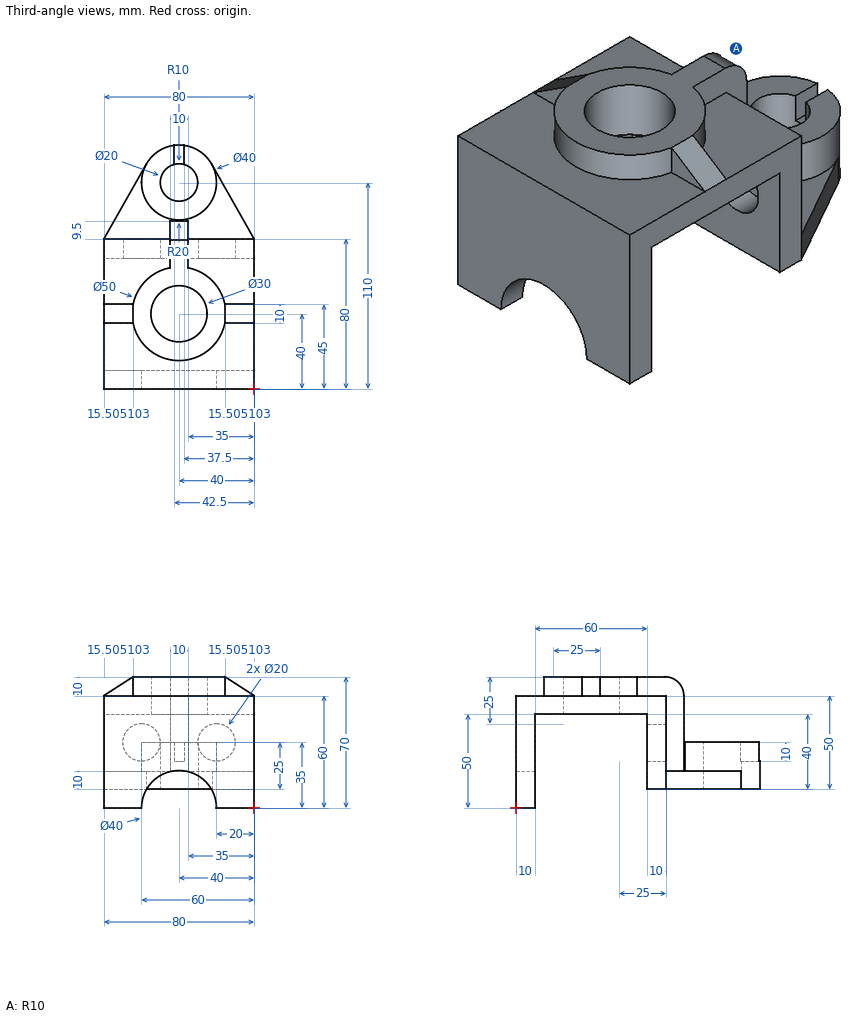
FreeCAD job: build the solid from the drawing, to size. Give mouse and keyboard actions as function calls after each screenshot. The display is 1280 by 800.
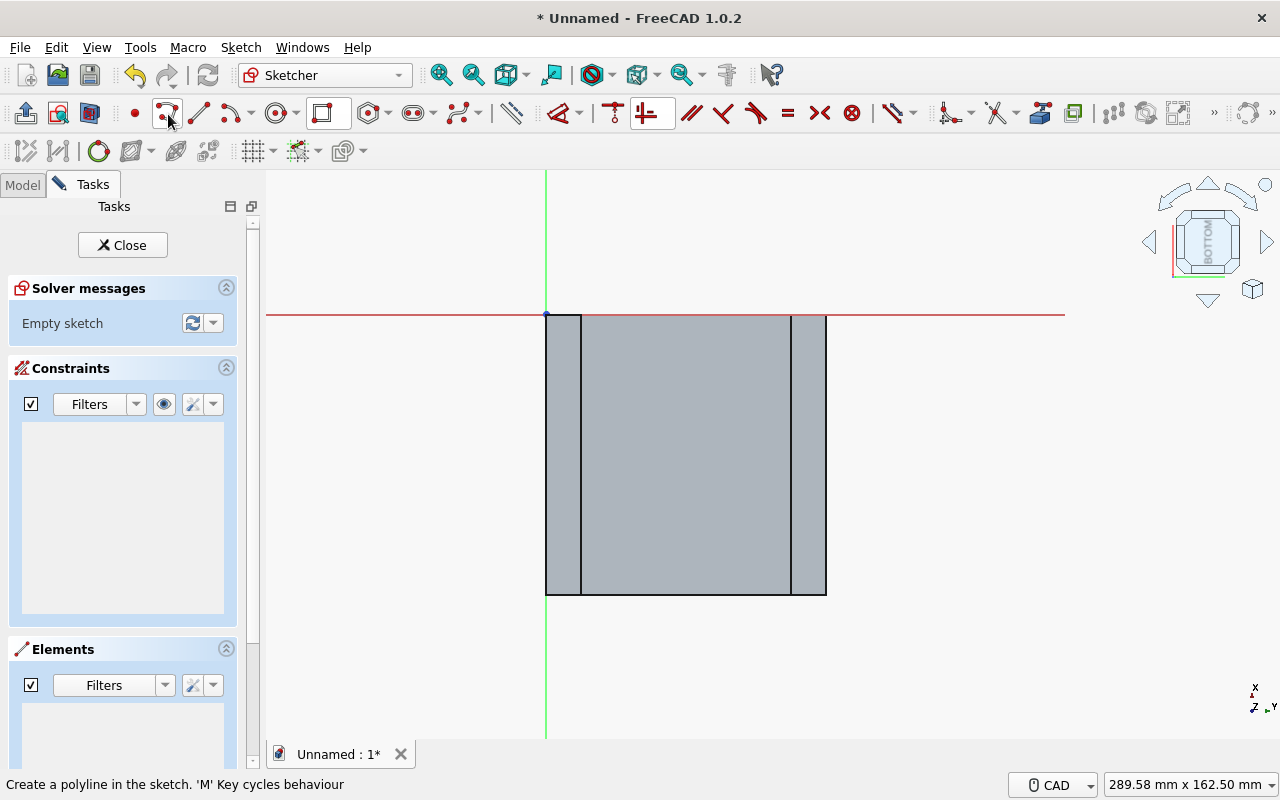
click(966, 394)
click(826, 315)
click(826, 595)
click(966, 516)
right_click(966, 516)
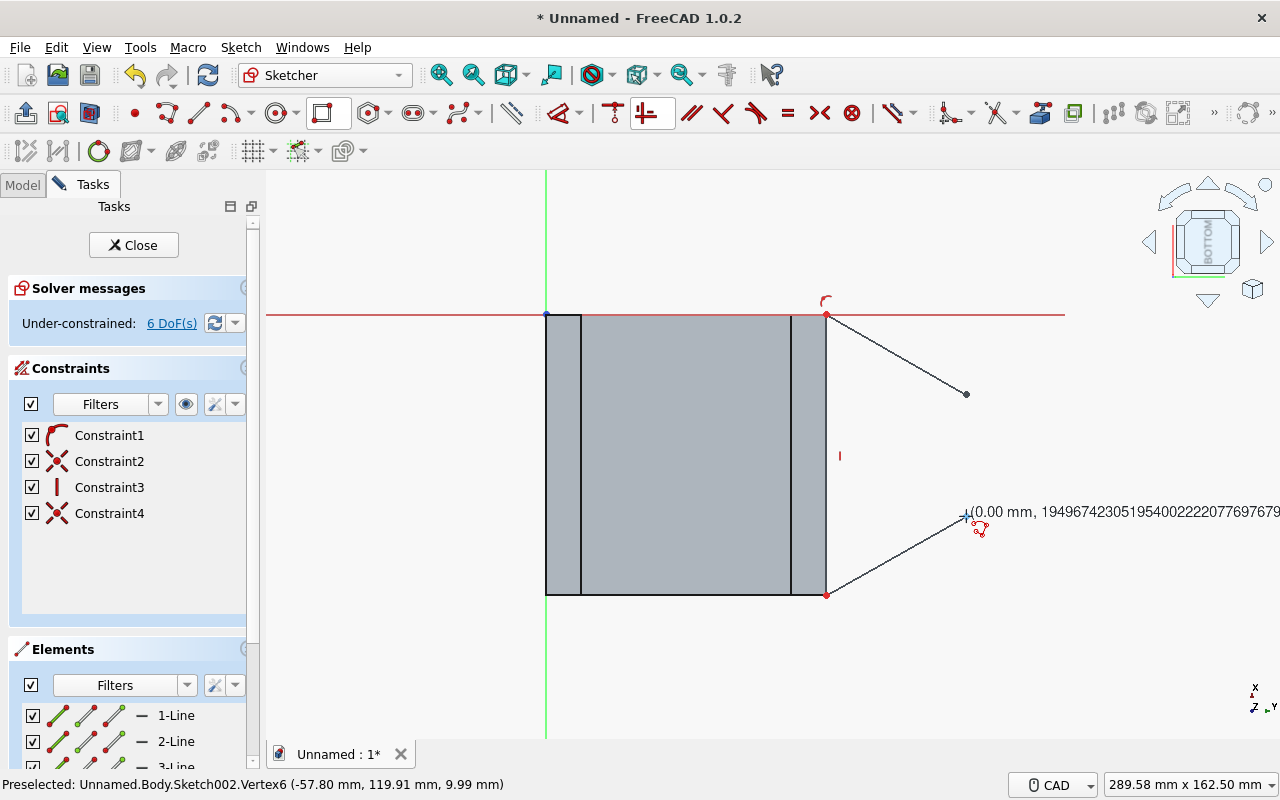
click(254, 114)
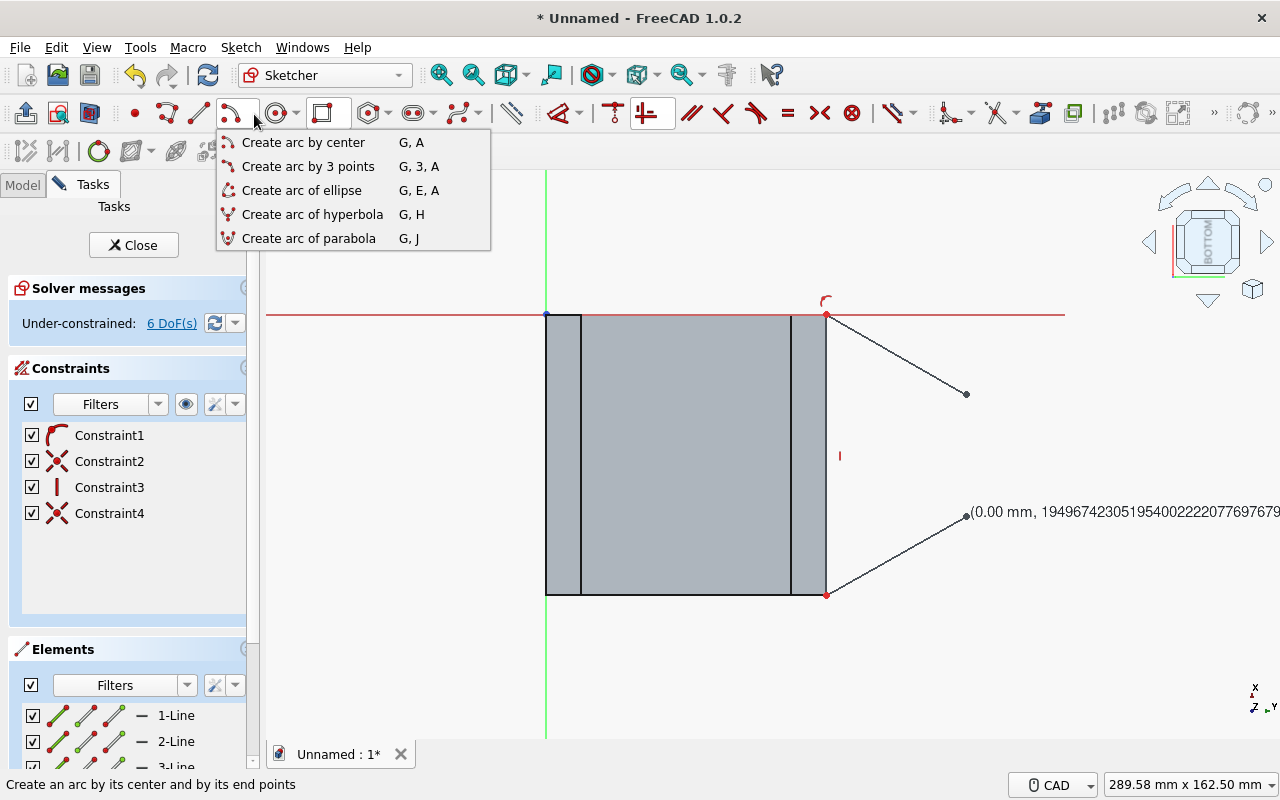
click(354, 166)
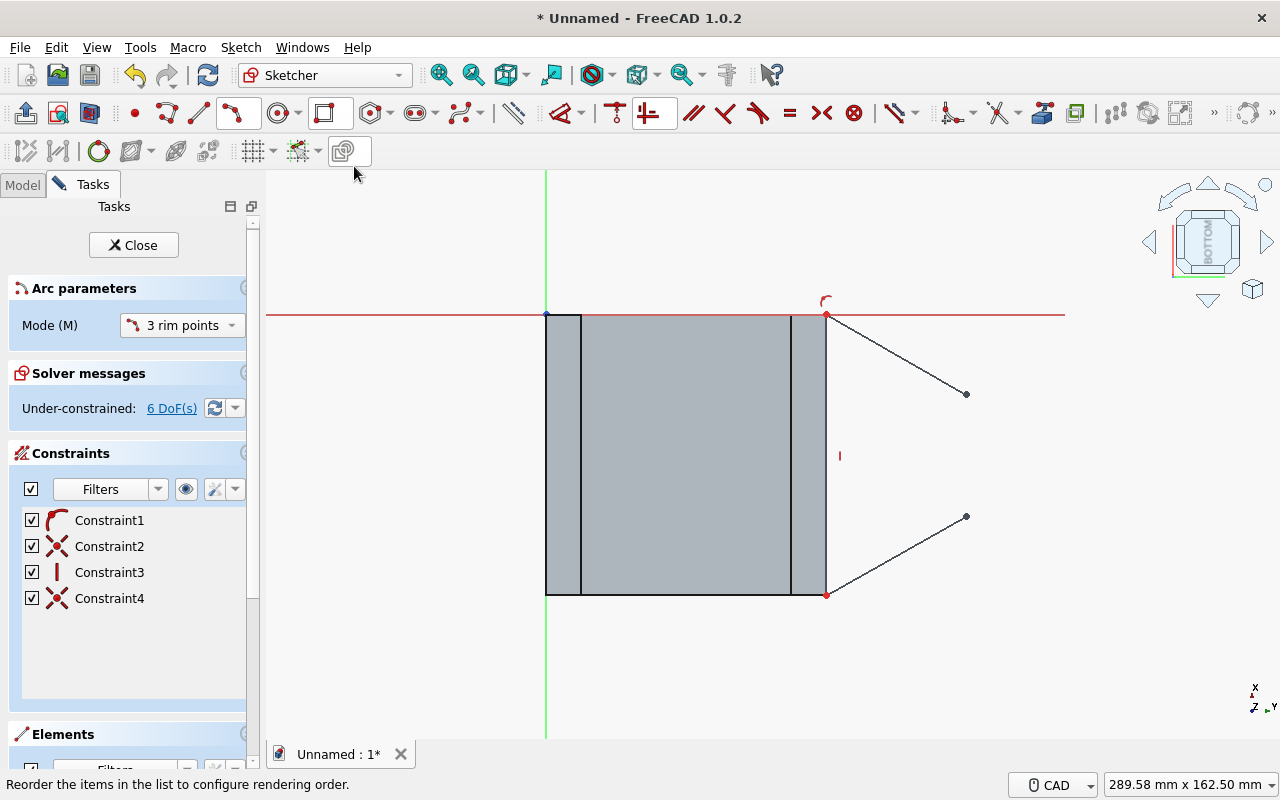
click(966, 517)
click(966, 395)
click(861, 455)
key(Escape)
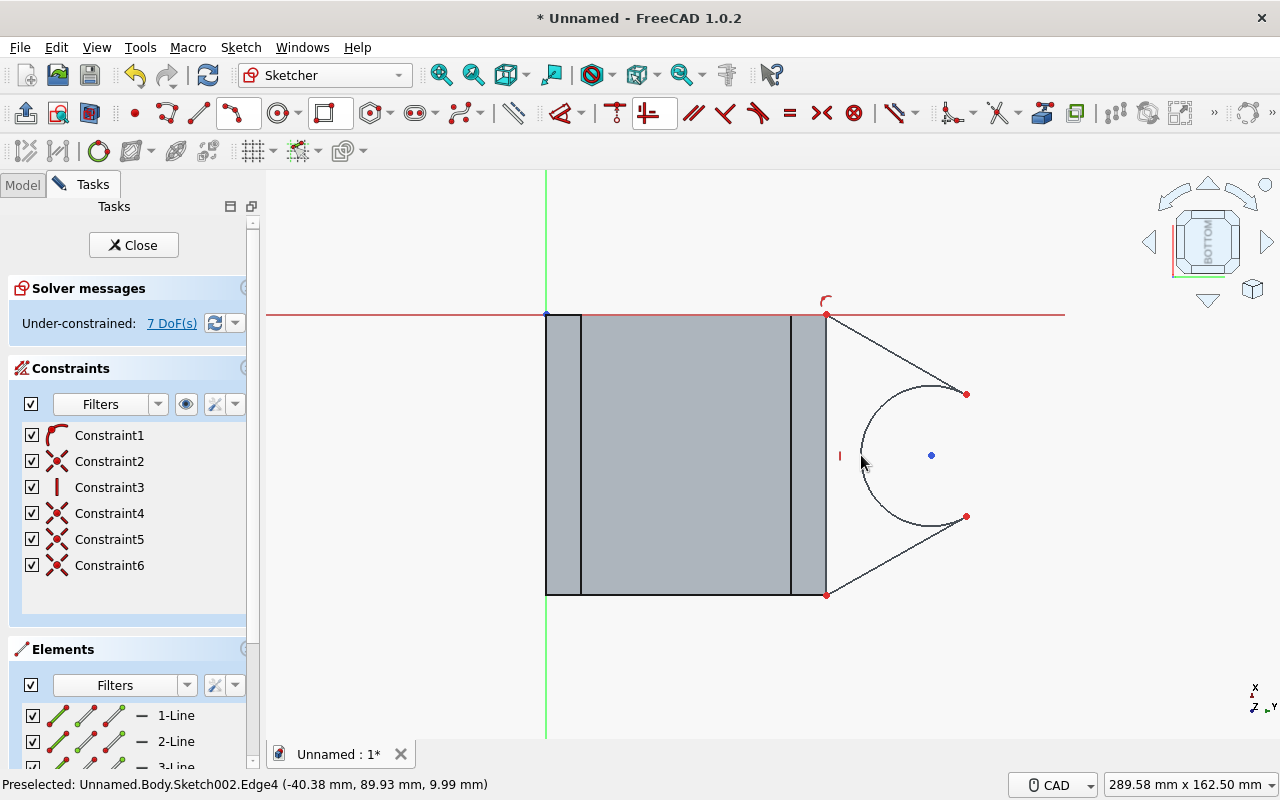
click(924, 371)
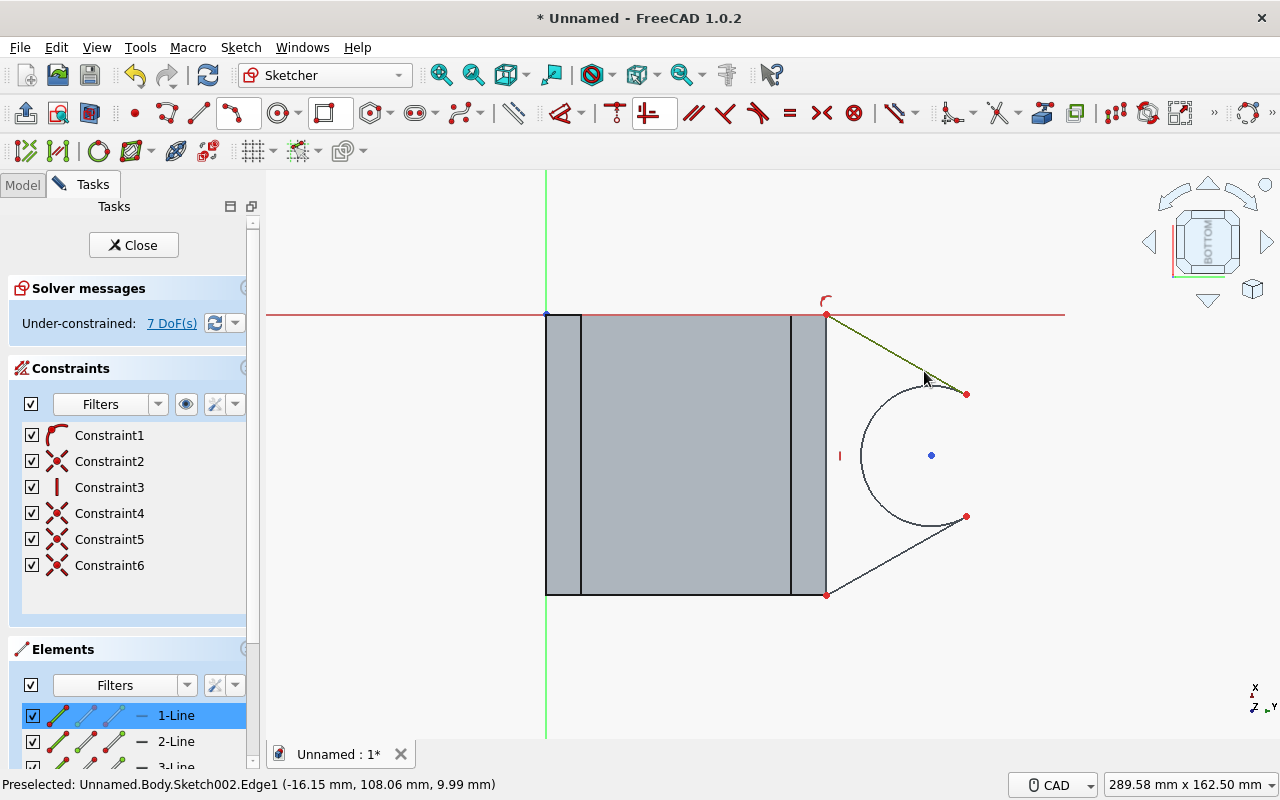
click(884, 404)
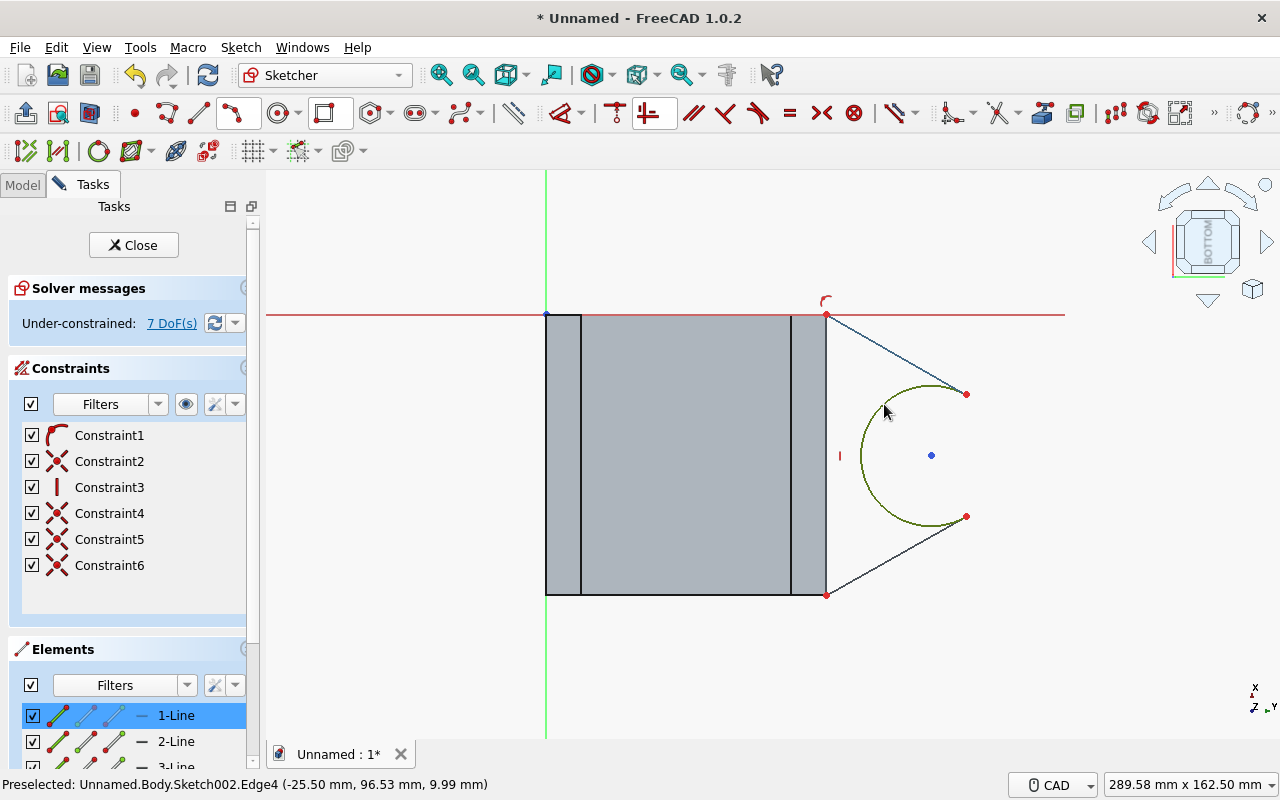
click(758, 114)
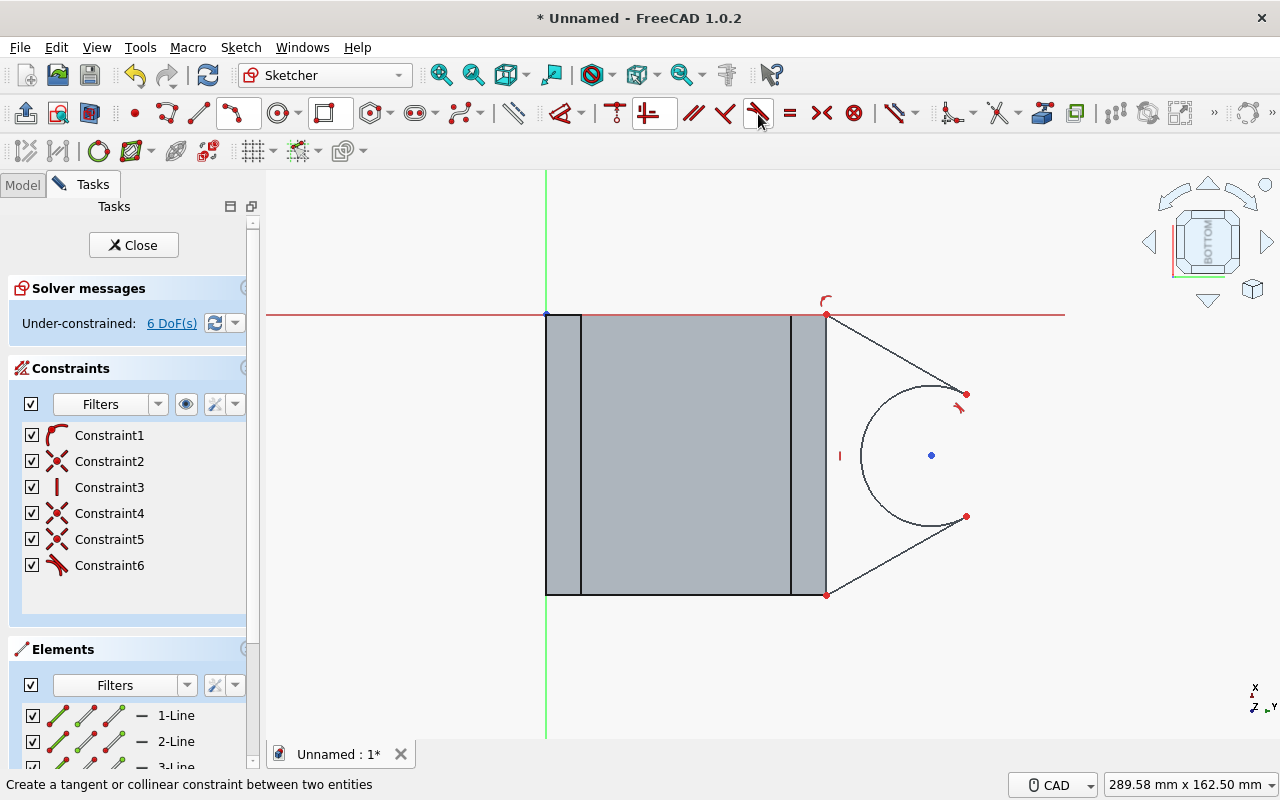
click(868, 572)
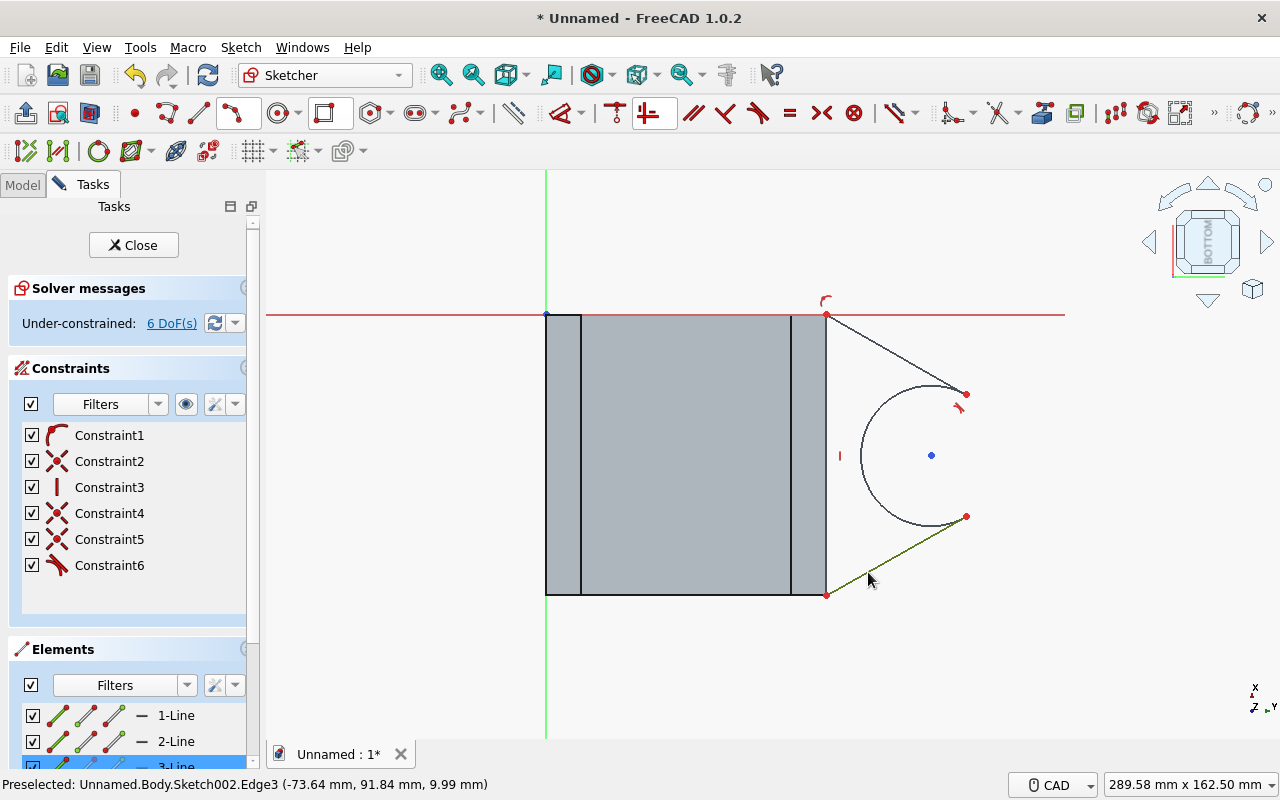
click(884, 404)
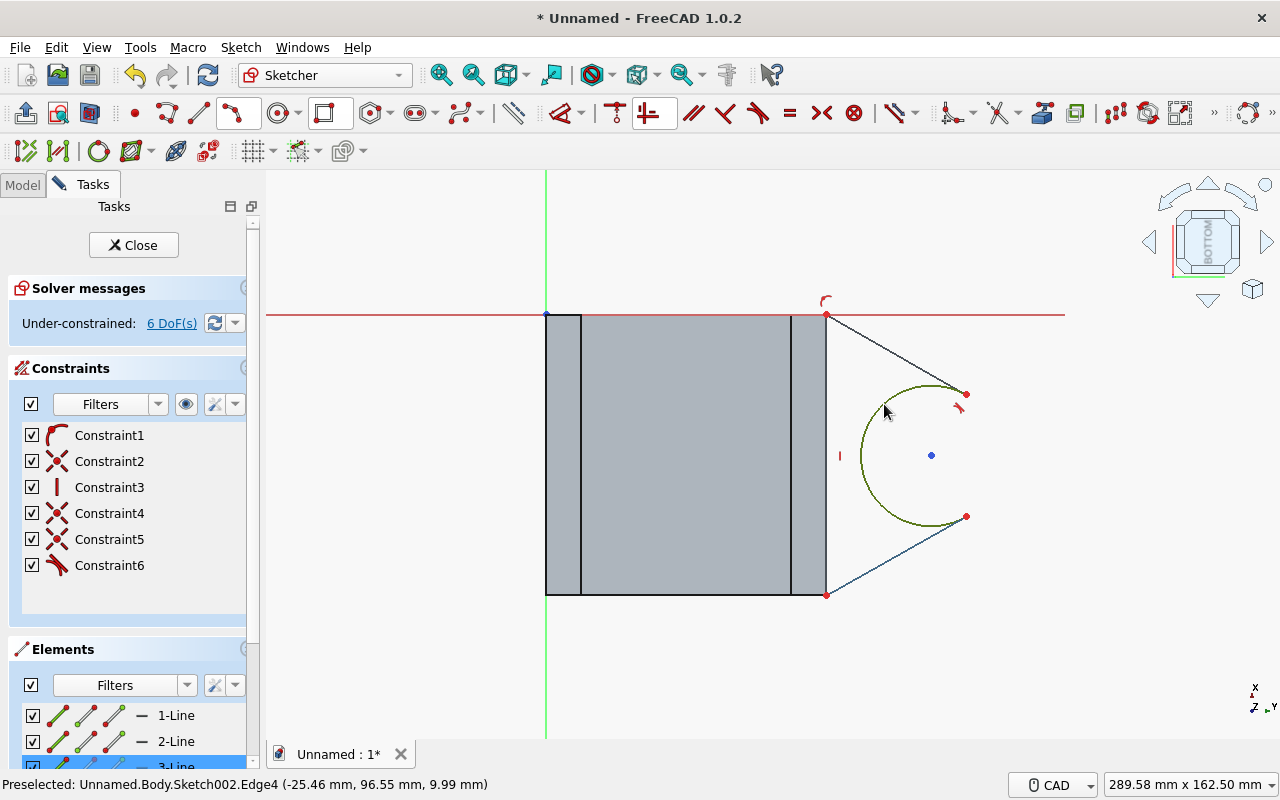
click(758, 114)